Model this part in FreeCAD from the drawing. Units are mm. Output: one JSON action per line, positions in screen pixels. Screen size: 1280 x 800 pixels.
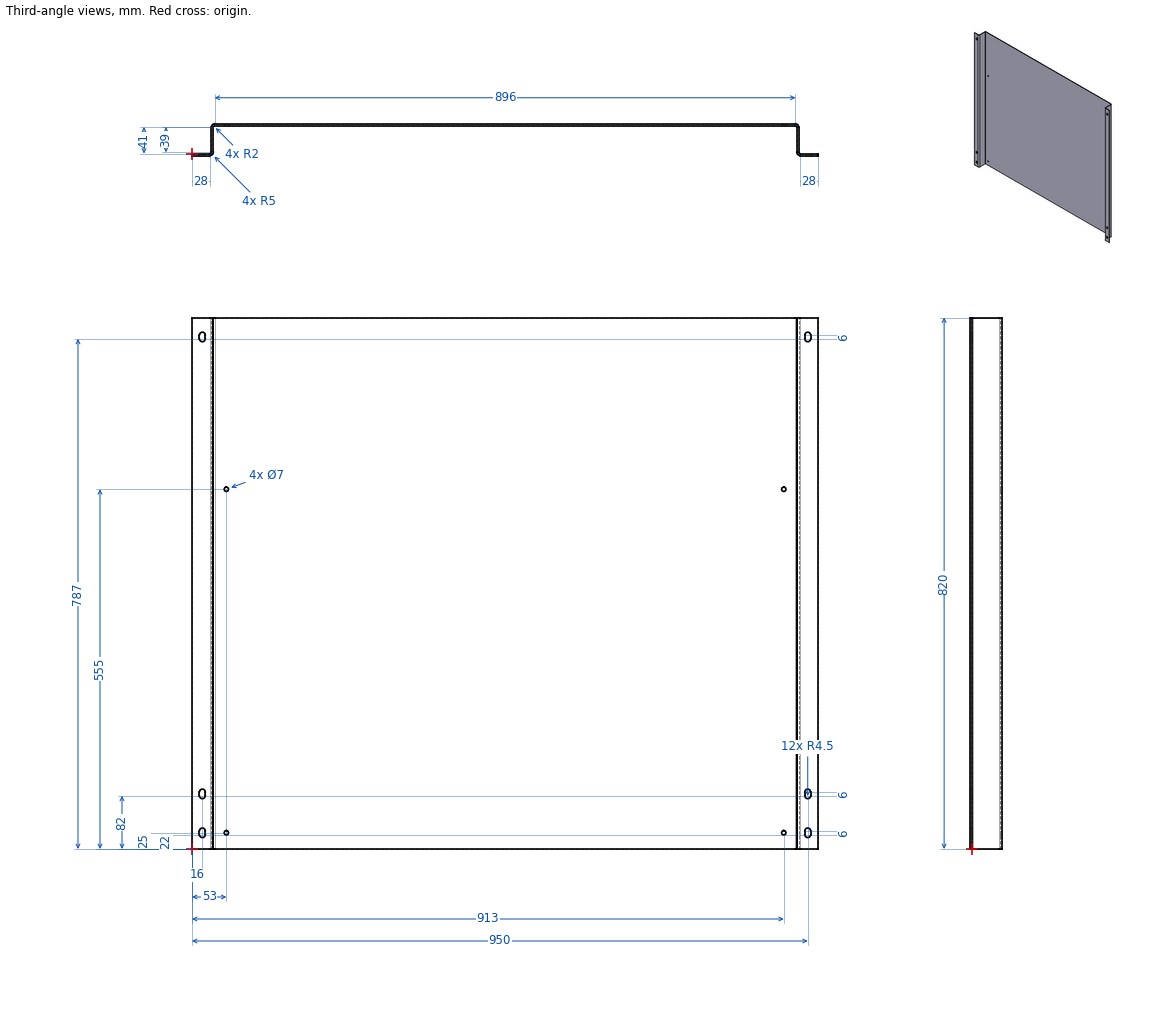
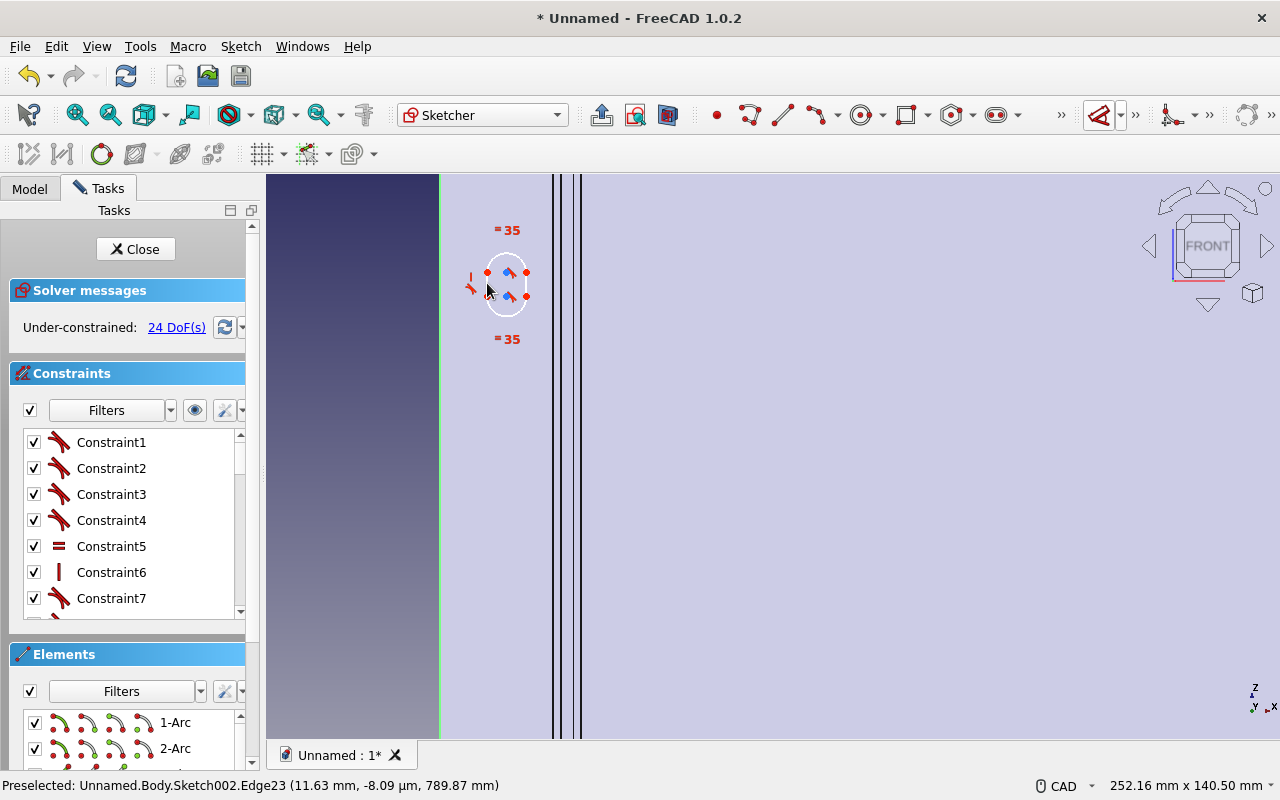
{"action": "scroll", "coordinate": [498, 282], "scroll_direction": "down", "scroll_amount": 11}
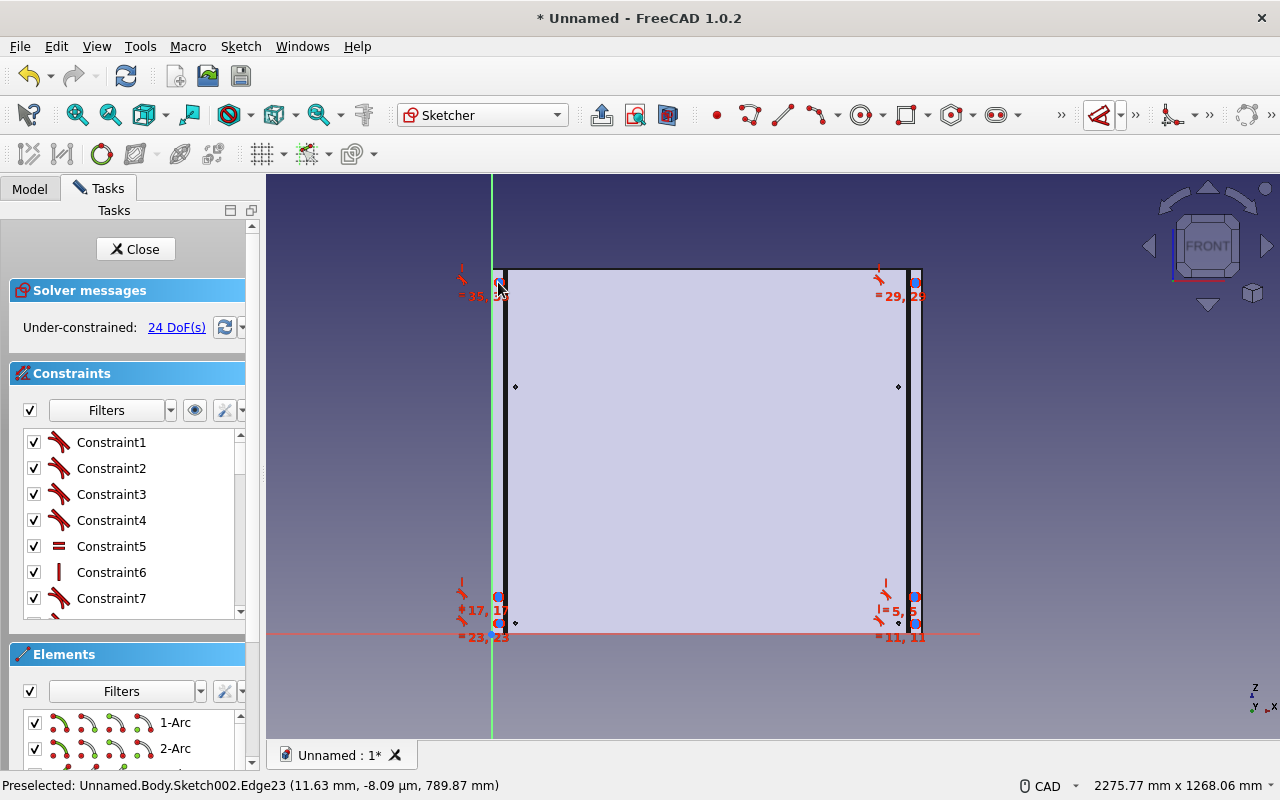
{"action": "scroll", "coordinate": [914, 601], "scroll_direction": "up", "scroll_amount": 10}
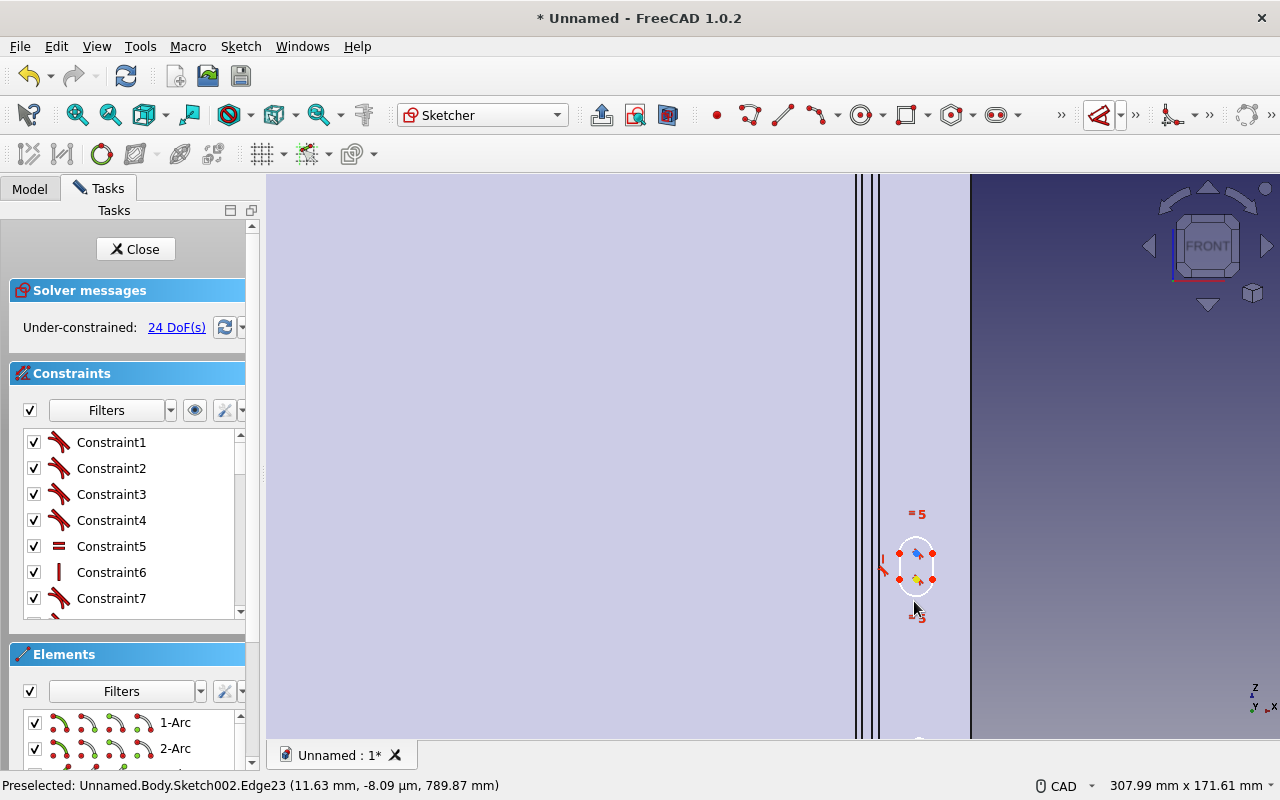
{"action": "left_click", "coordinate": [906, 593]}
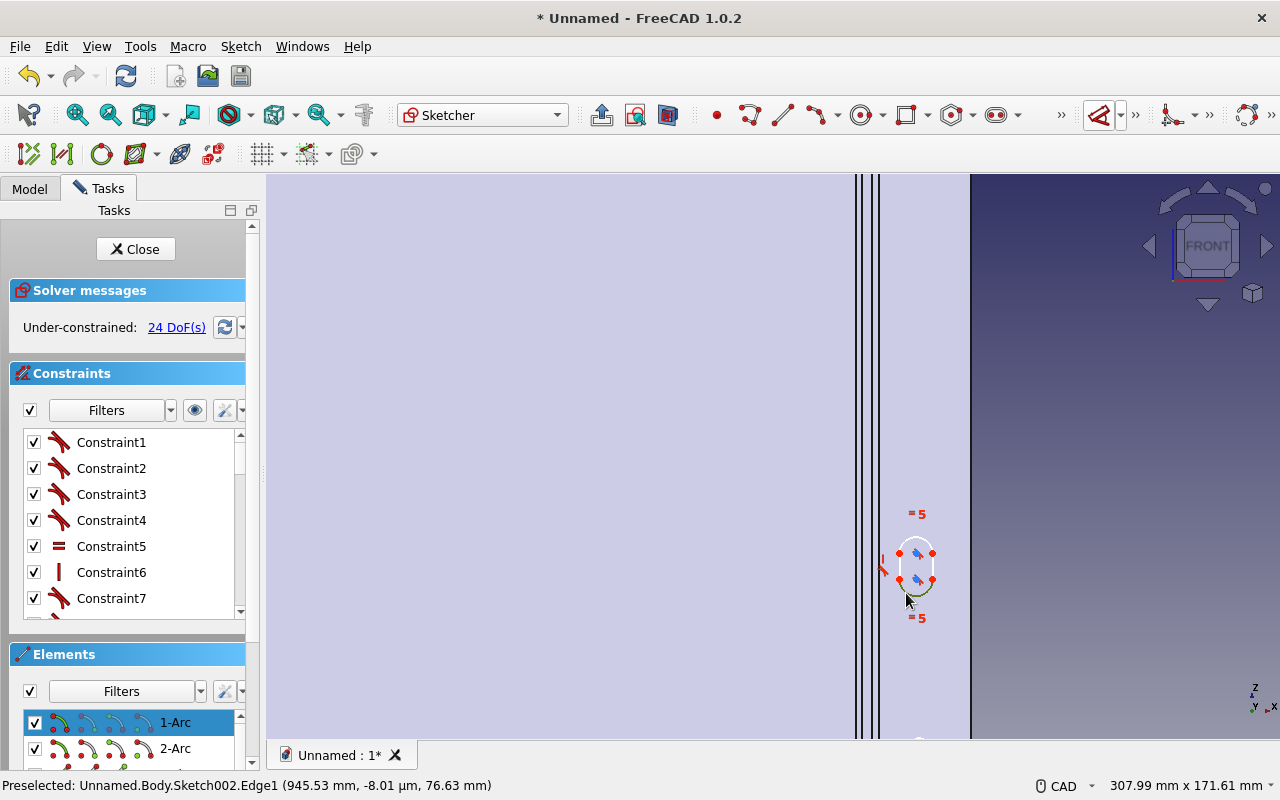
{"action": "scroll", "coordinate": [915, 602], "scroll_direction": "down", "scroll_amount": 10}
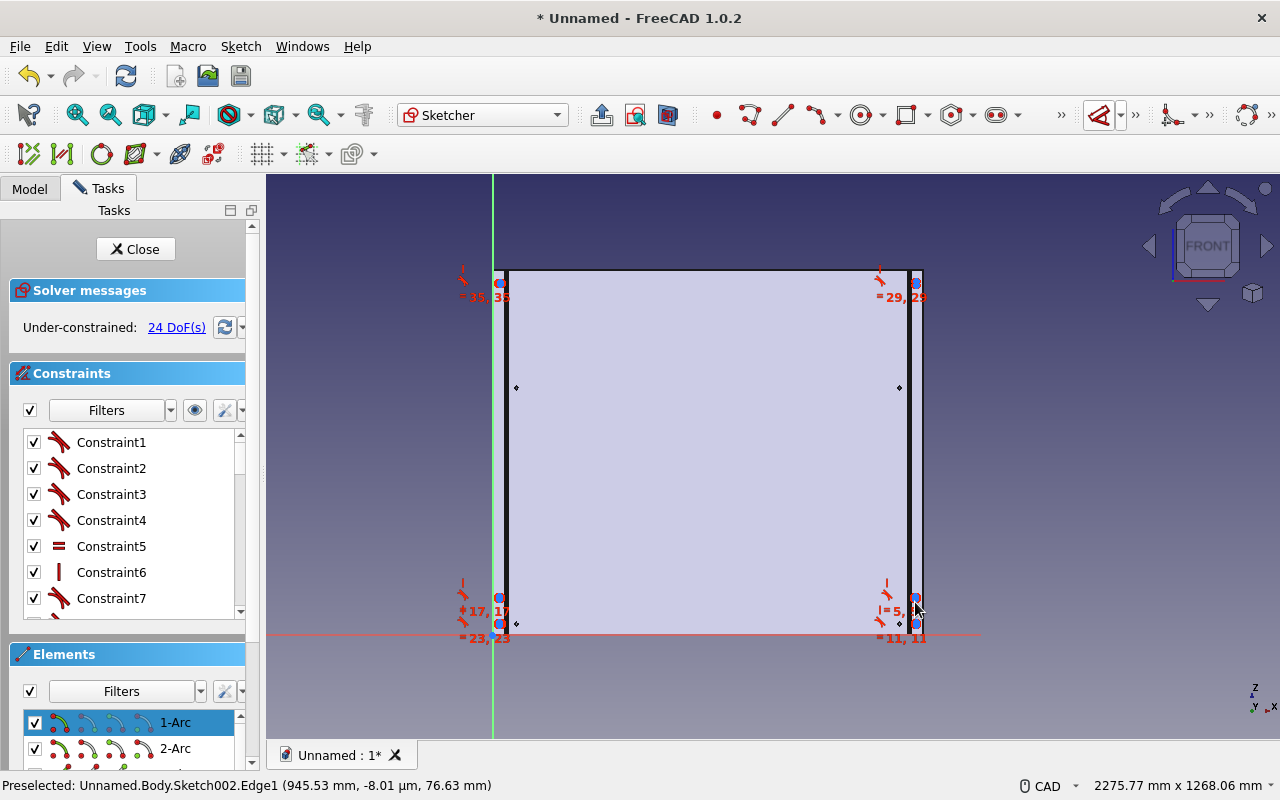
{"action": "scroll", "coordinate": [915, 627], "scroll_direction": "up", "scroll_amount": 11}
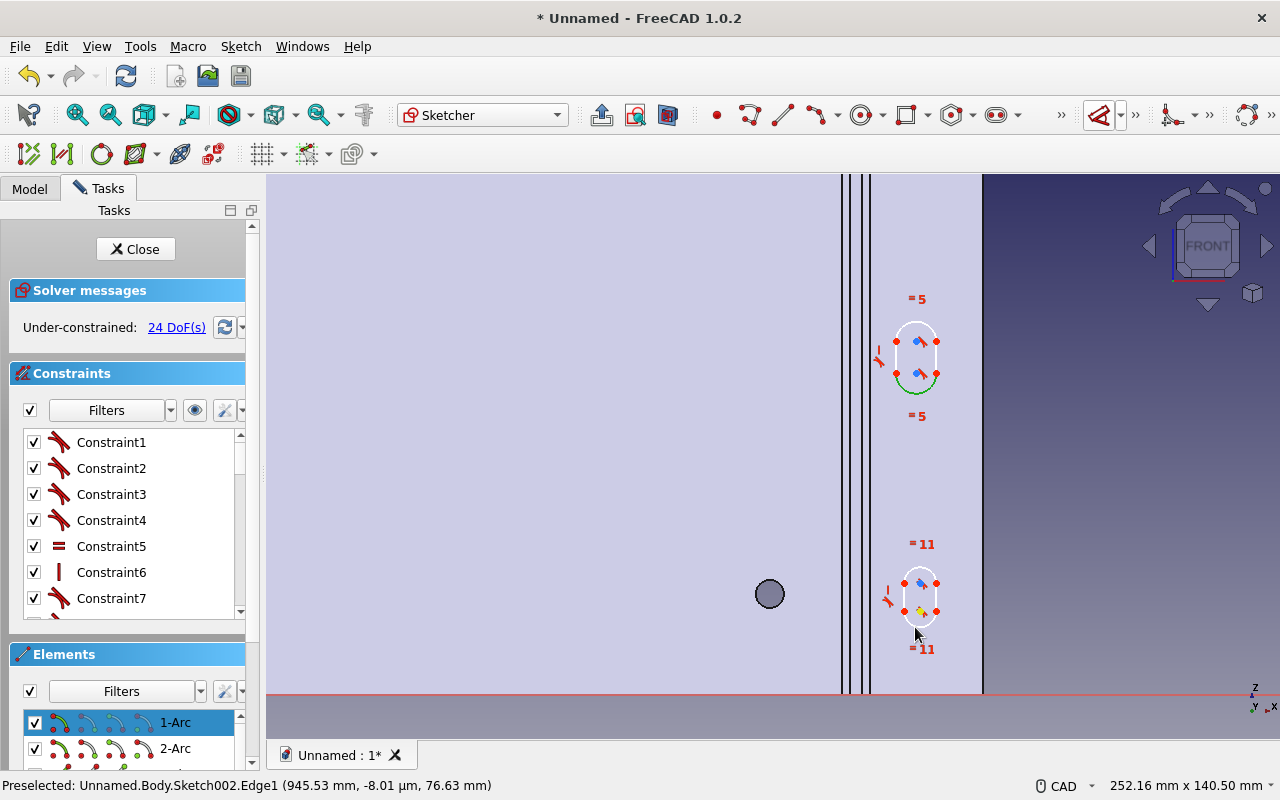
{"action": "left_click", "coordinate": [911, 624]}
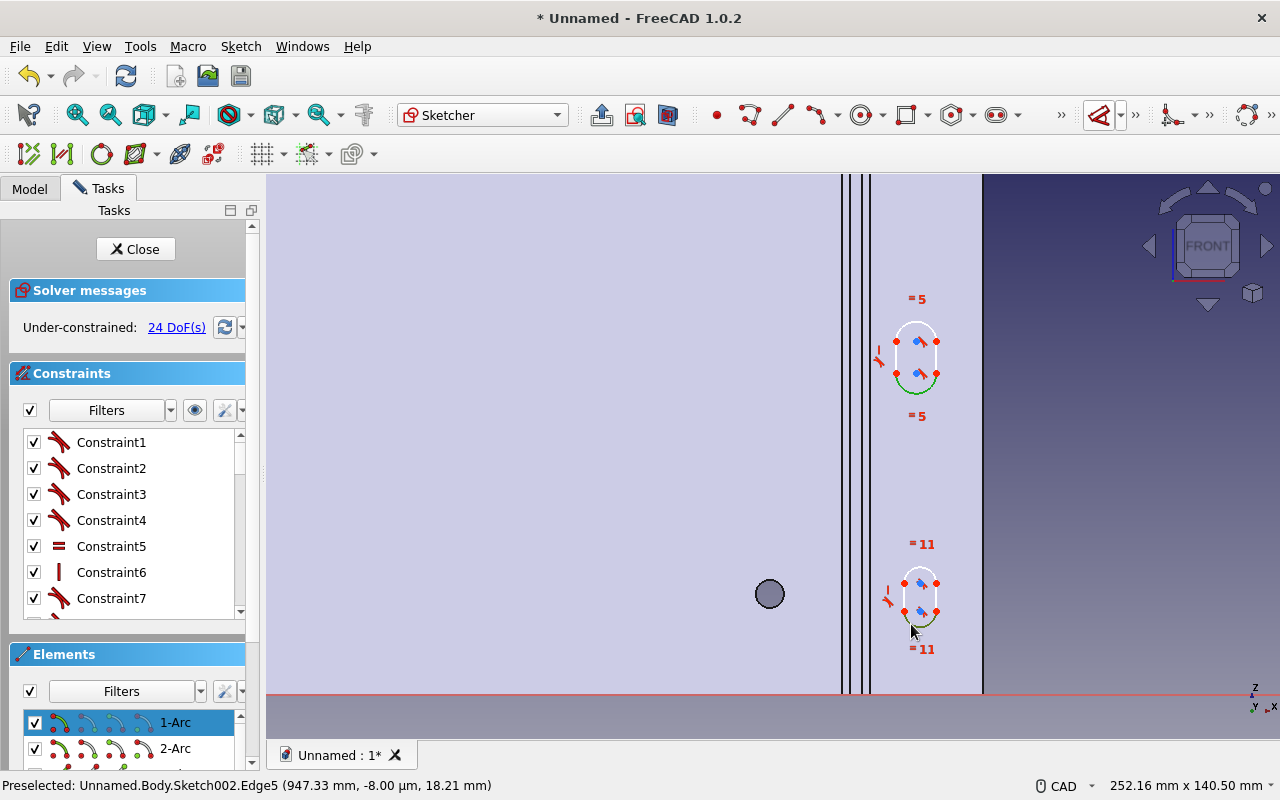
{"action": "scroll", "coordinate": [915, 627], "scroll_direction": "down", "scroll_amount": 11}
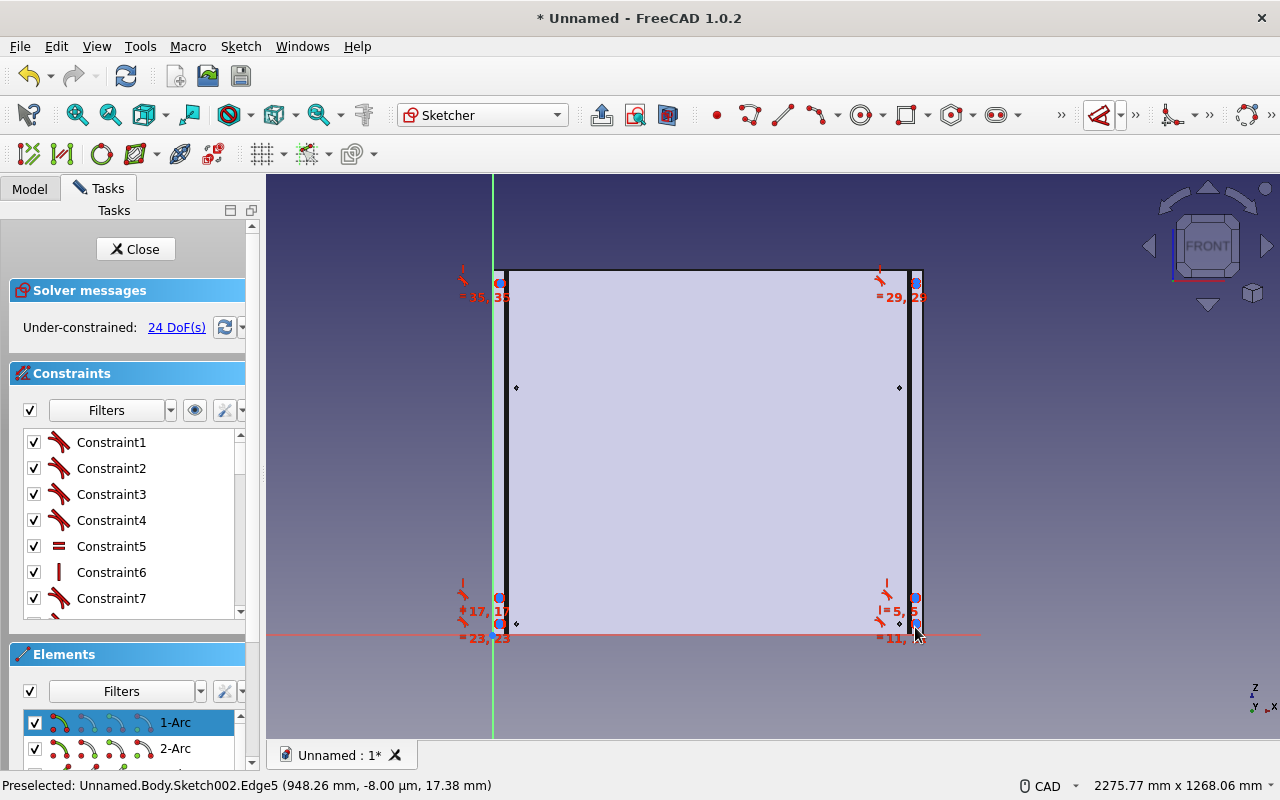
{"action": "scroll", "coordinate": [499, 601], "scroll_direction": "up", "scroll_amount": 11}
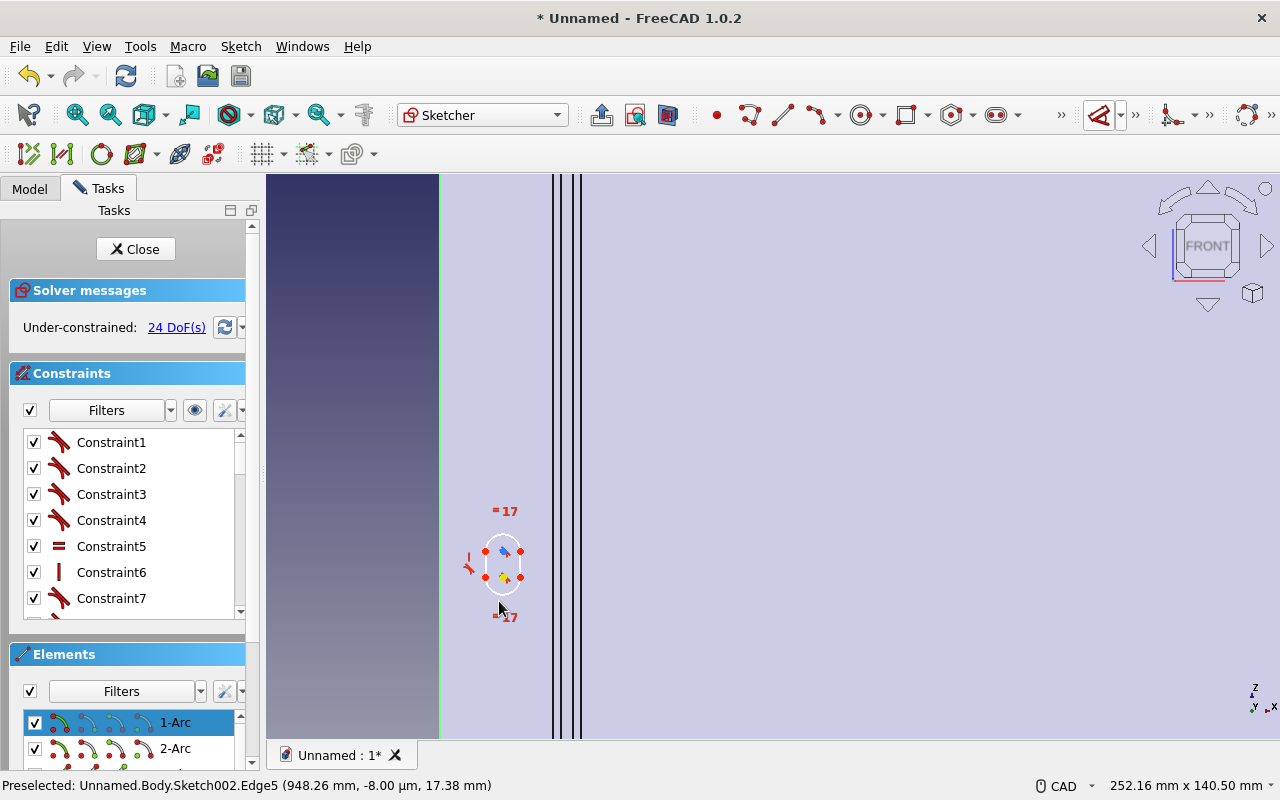
{"action": "left_click", "coordinate": [493, 591]}